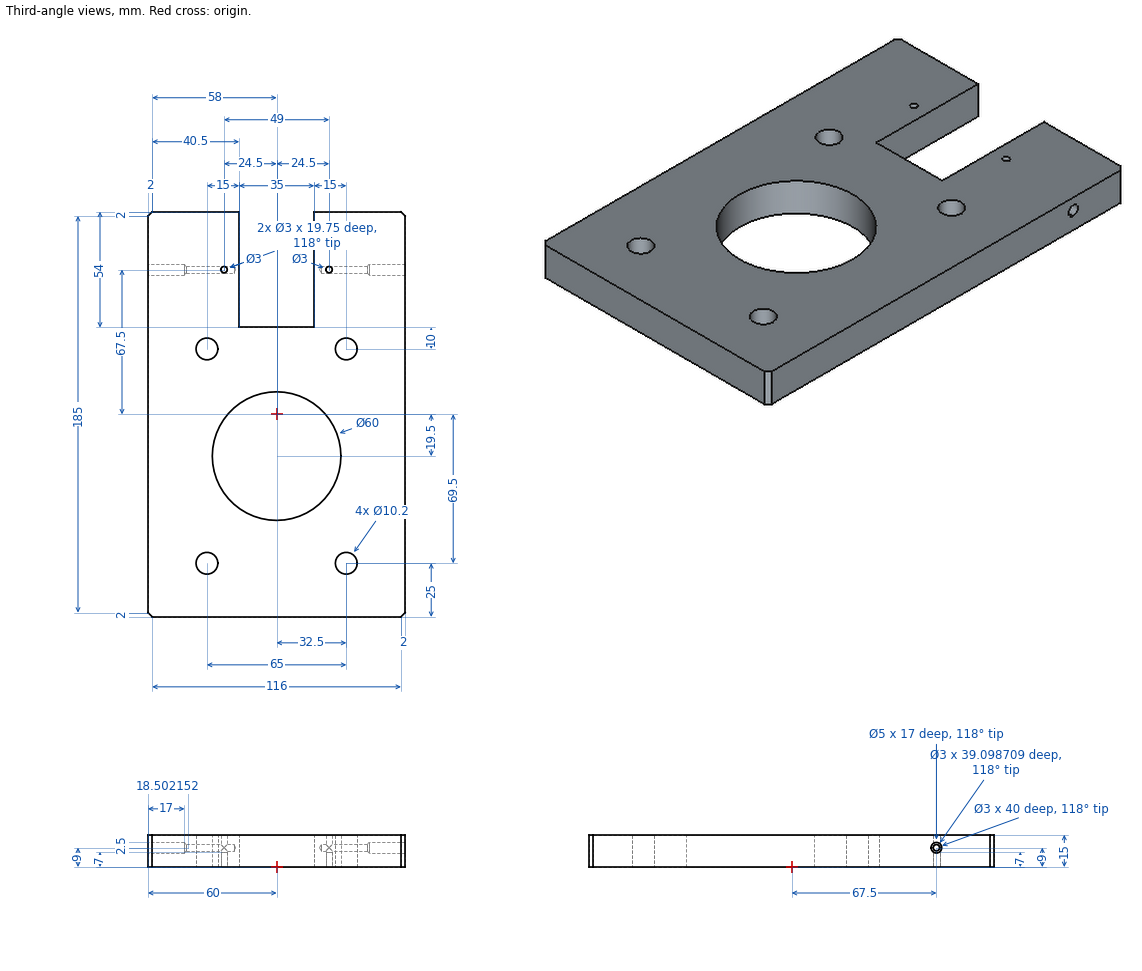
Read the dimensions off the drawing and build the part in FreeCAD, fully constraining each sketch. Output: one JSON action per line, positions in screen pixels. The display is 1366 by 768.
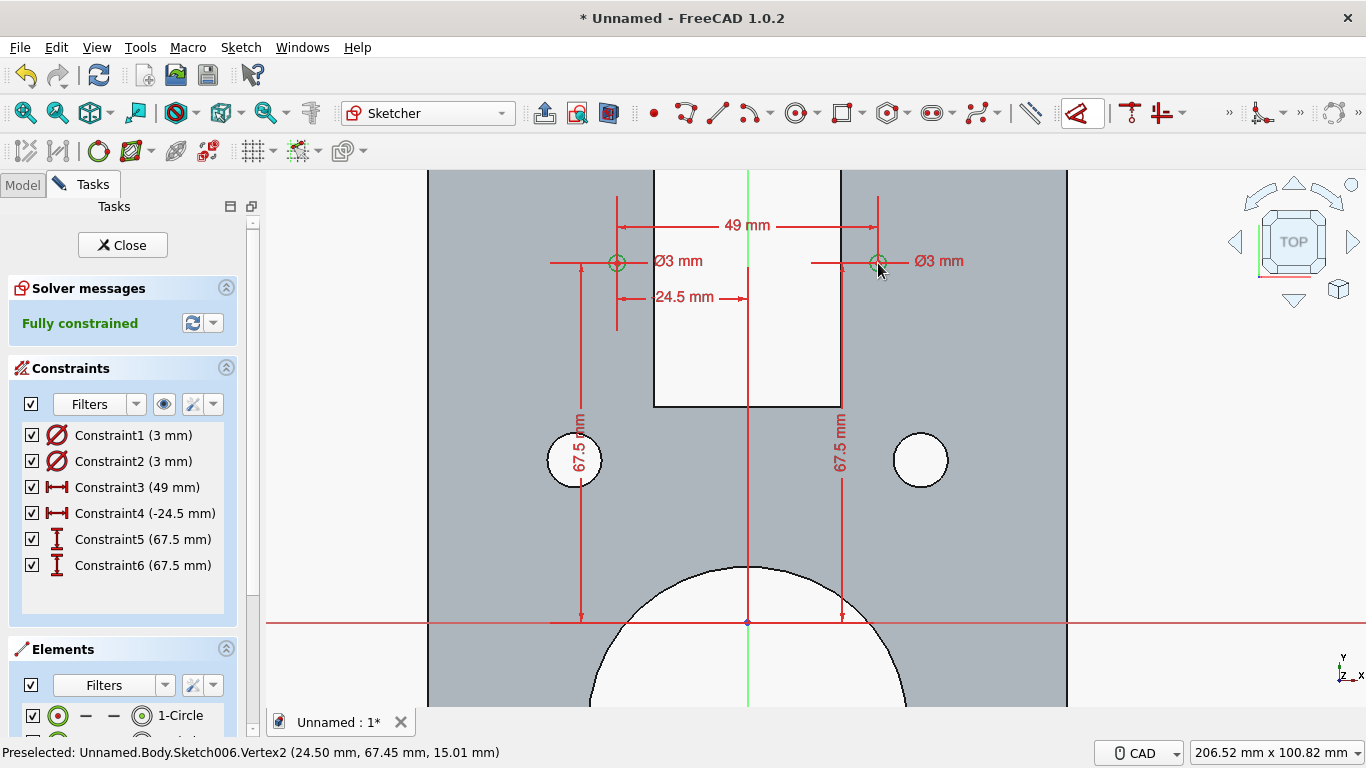
{"action": "left_click", "coordinate": [123, 245]}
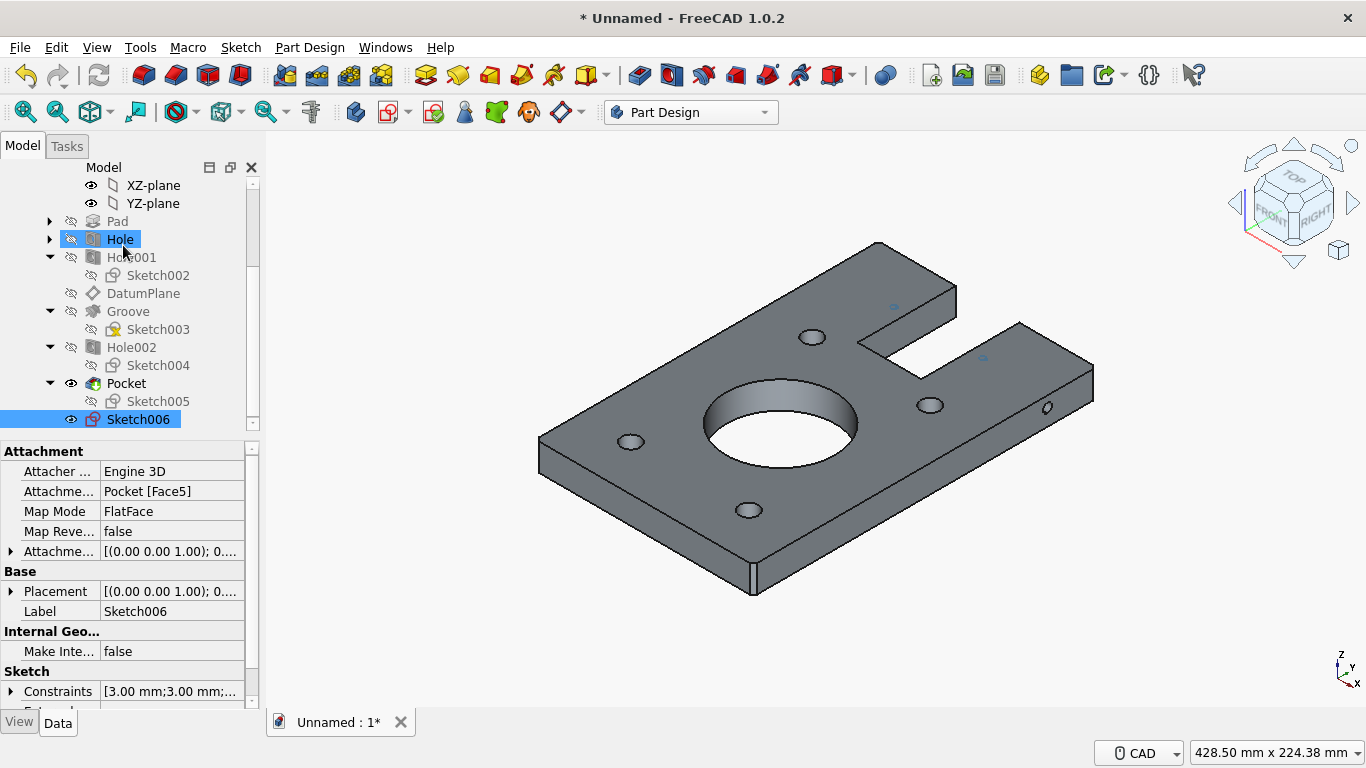
{"action": "left_click", "coordinate": [672, 76]}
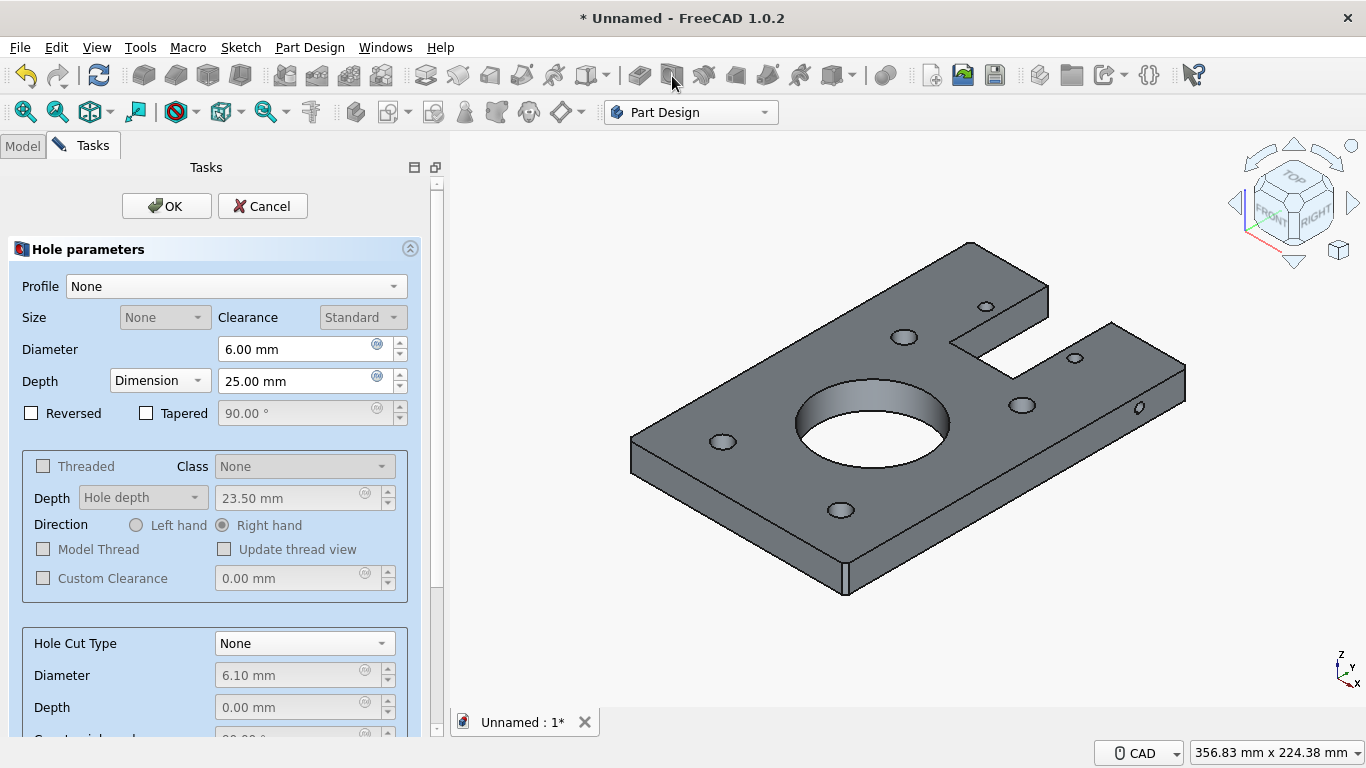
{"action": "triple_click", "coordinate": [305, 349]}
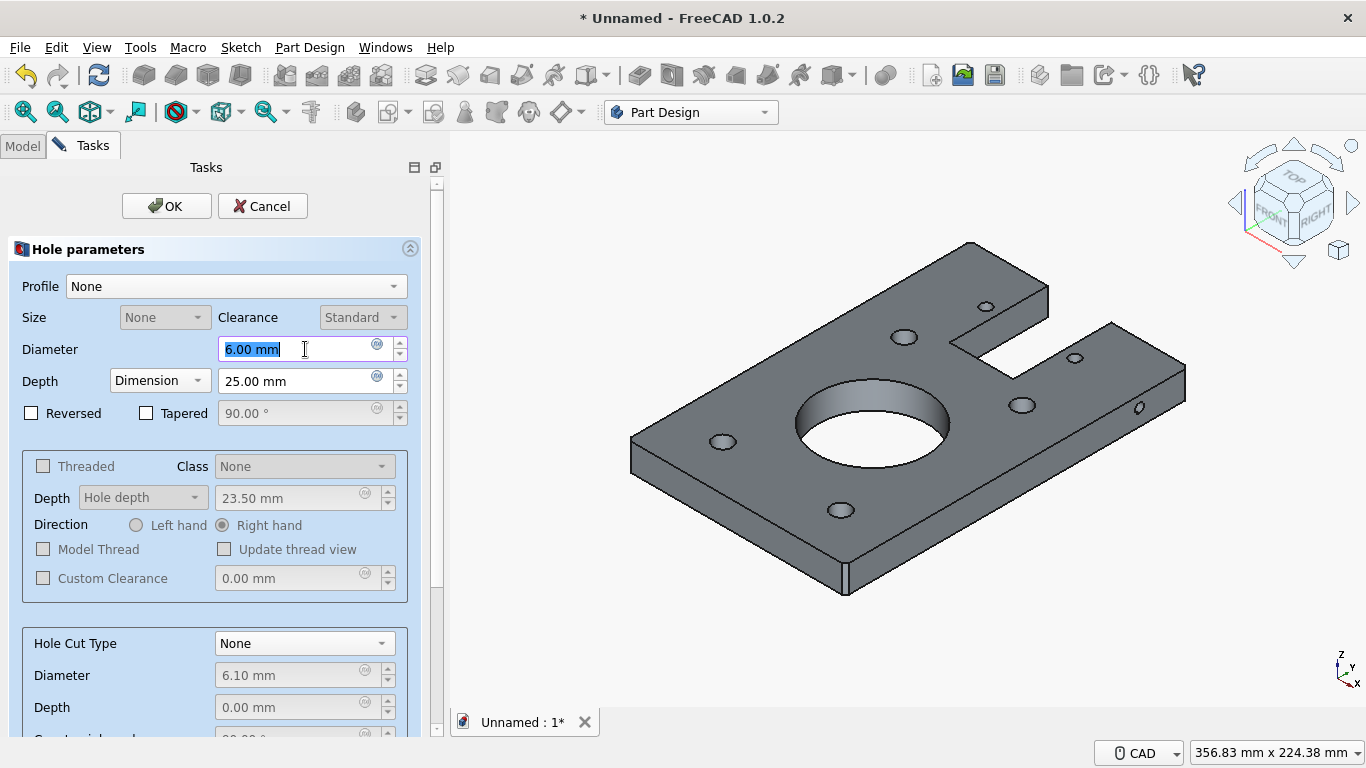
{"action": "type", "text": "3"}
{"action": "key", "text": "Tab"}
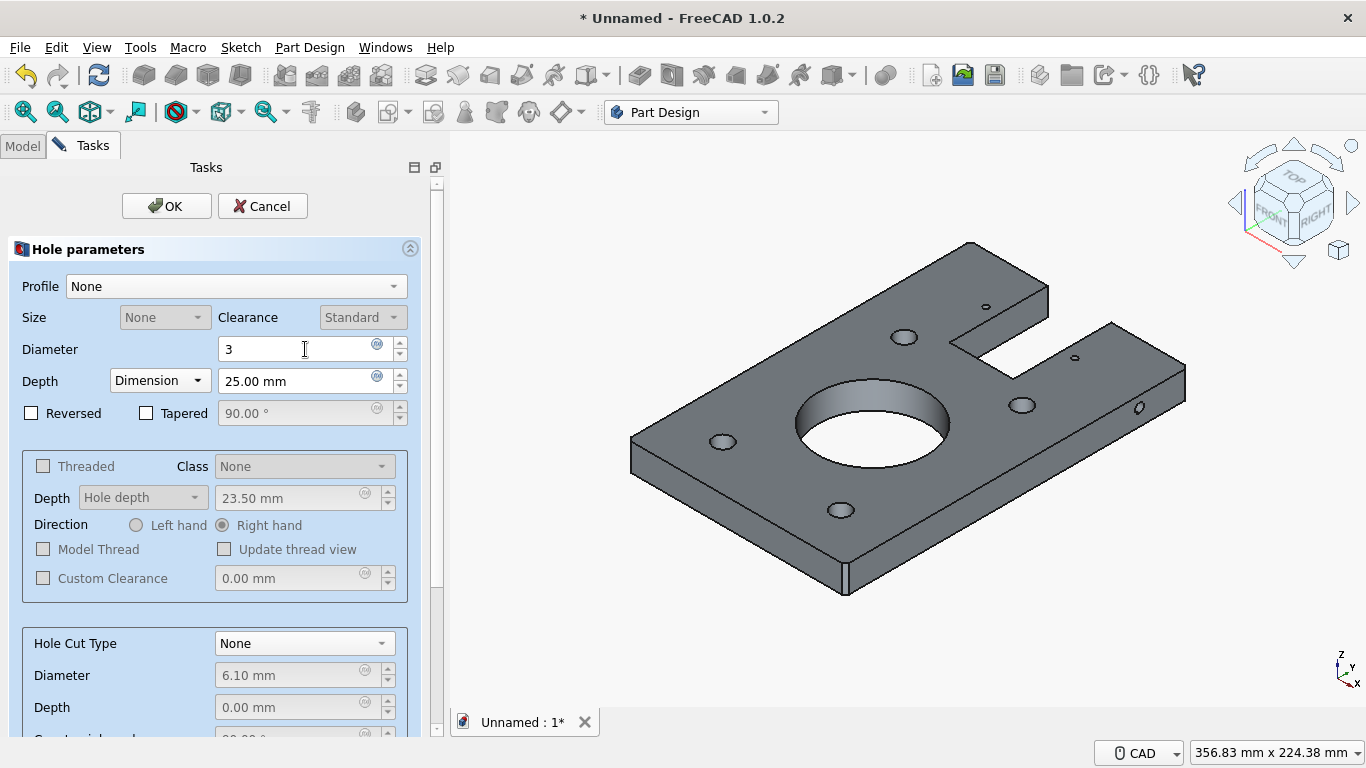
{"action": "triple_click", "coordinate": [305, 381]}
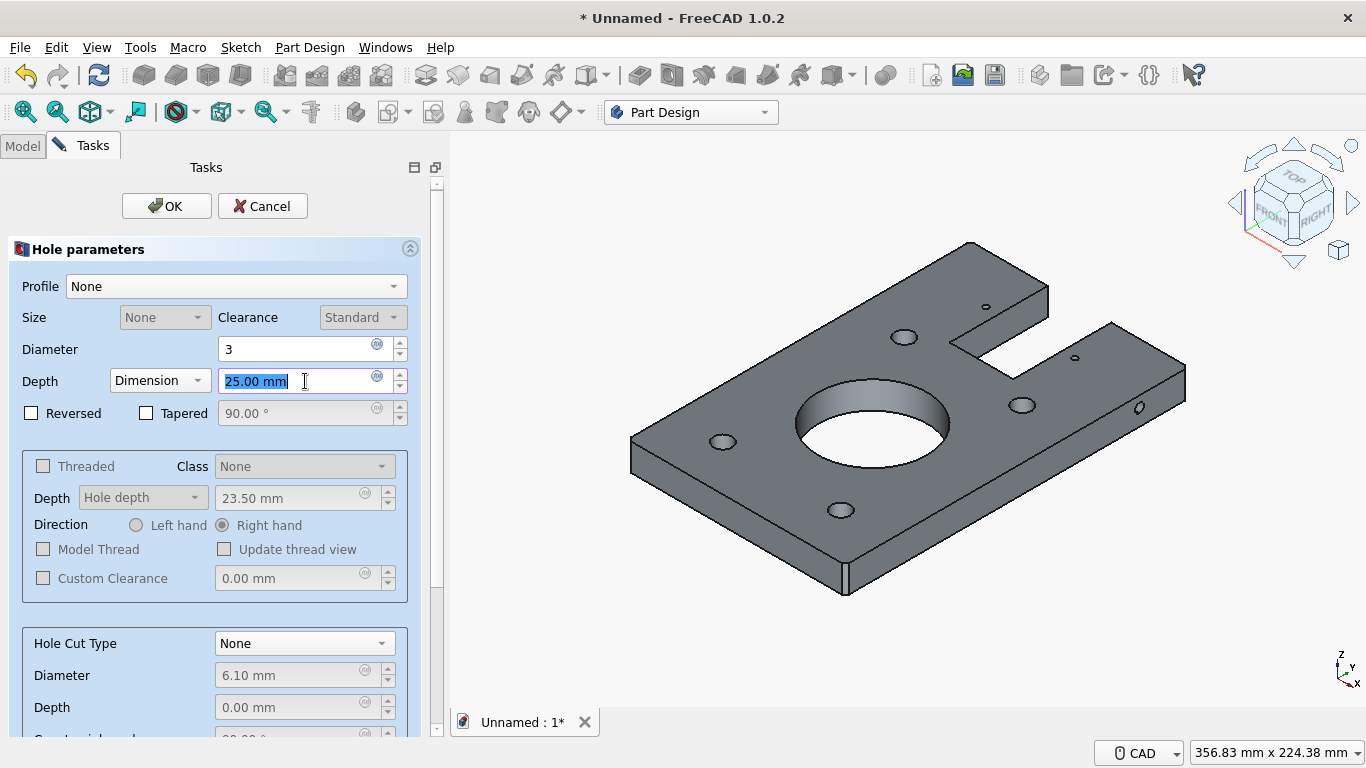
{"action": "type", "text": "19.75"}
{"action": "key", "text": "Tab"}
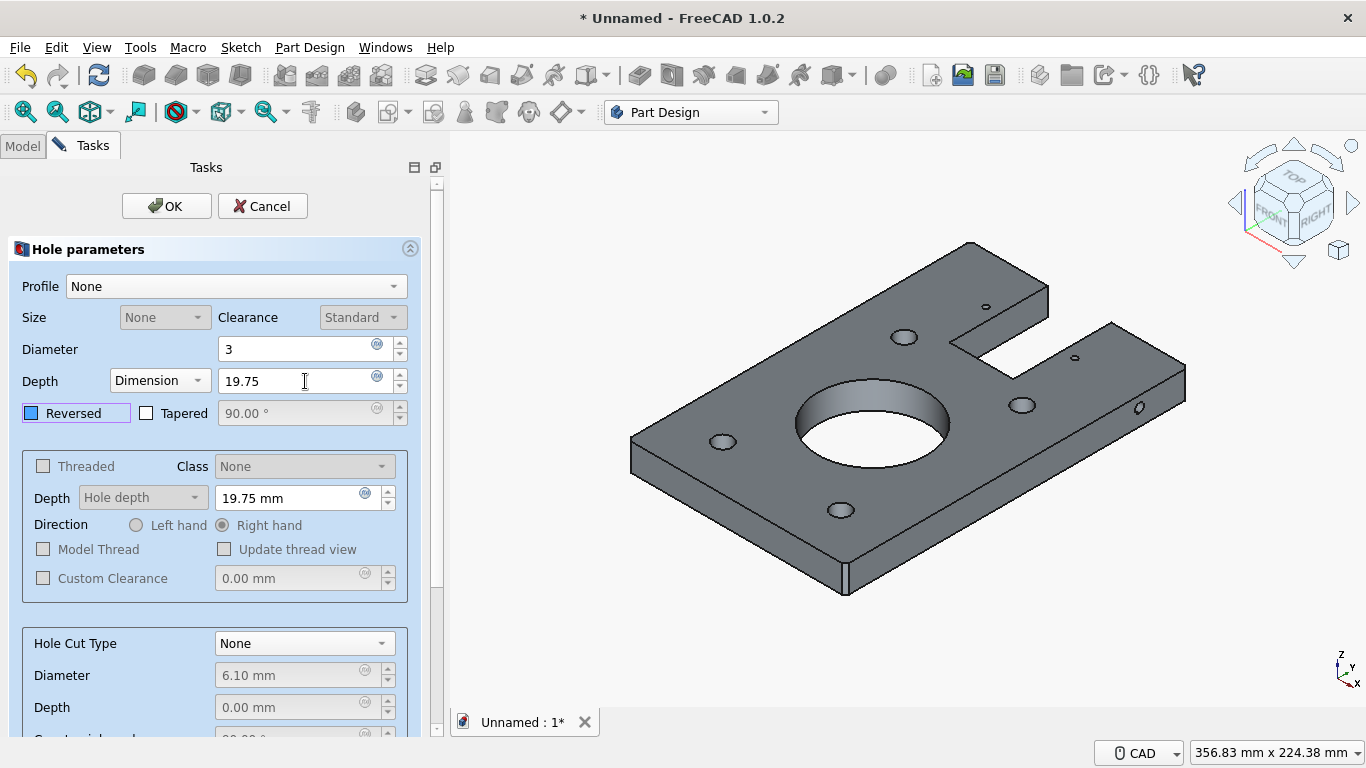
{"action": "left_click", "coordinate": [167, 206]}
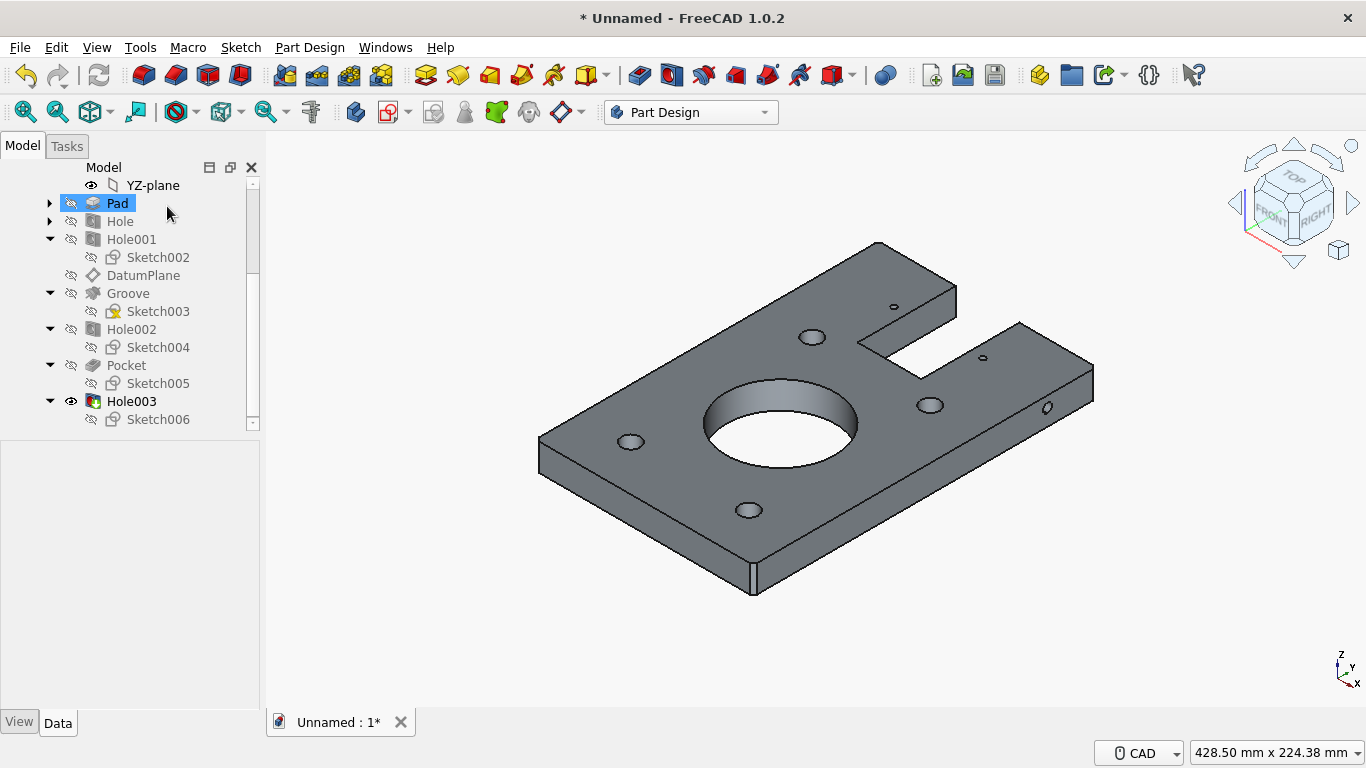
{"action": "left_click", "coordinate": [356, 112]}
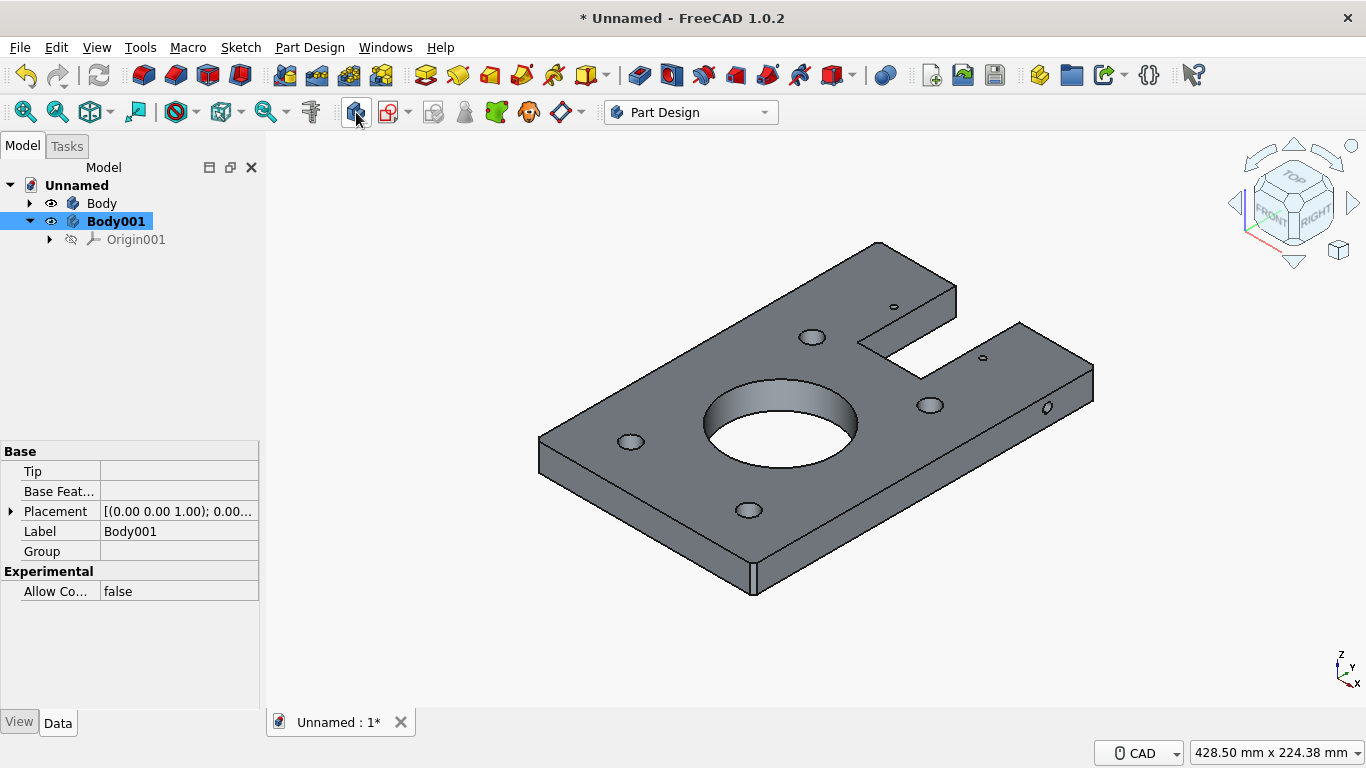
{"action": "left_click", "coordinate": [306, 667]}